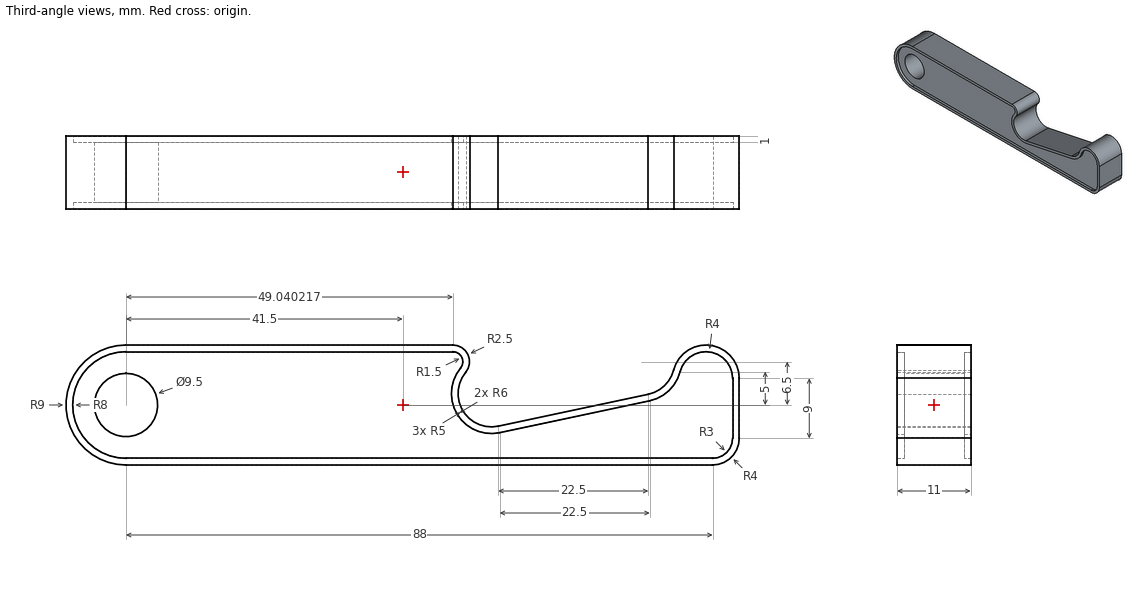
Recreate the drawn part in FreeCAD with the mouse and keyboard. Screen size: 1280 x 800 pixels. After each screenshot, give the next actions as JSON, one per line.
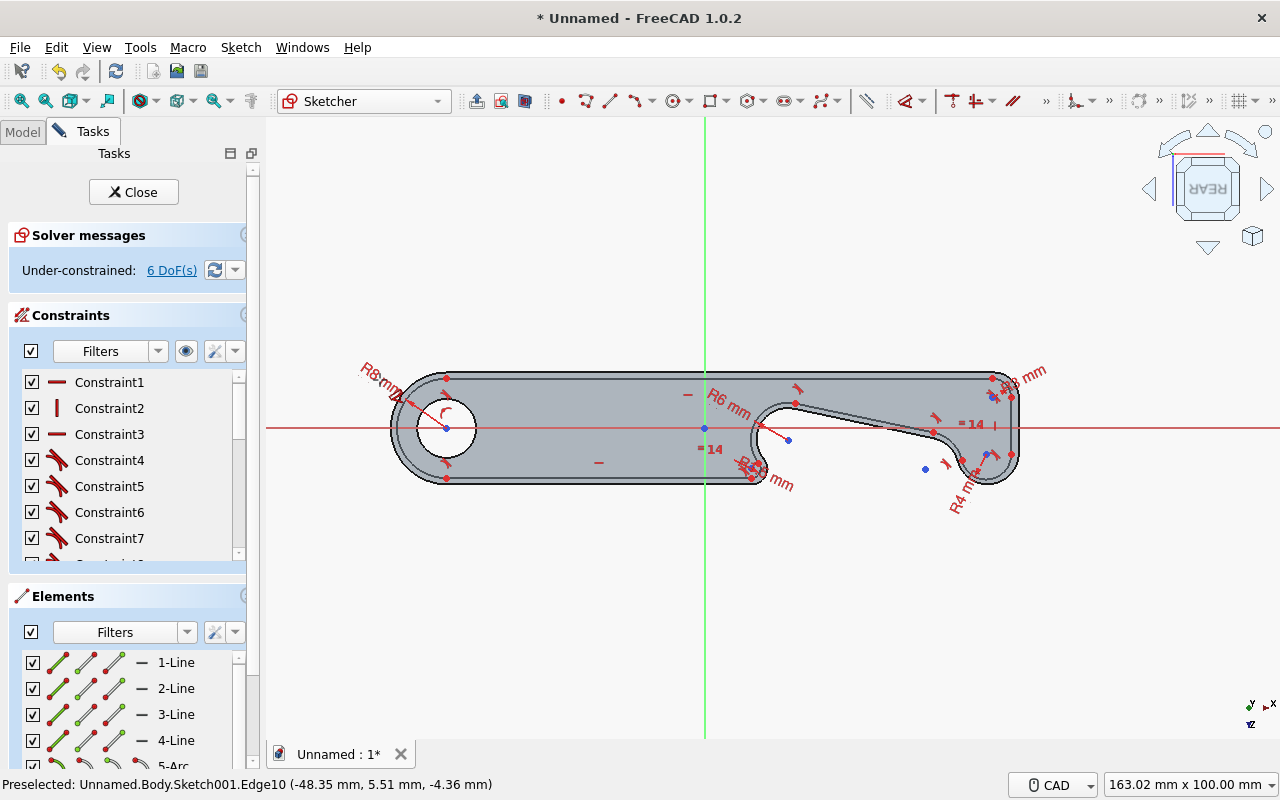
{"action": "scroll", "coordinate": [1011, 437], "scroll_direction": "up", "scroll_amount": 3}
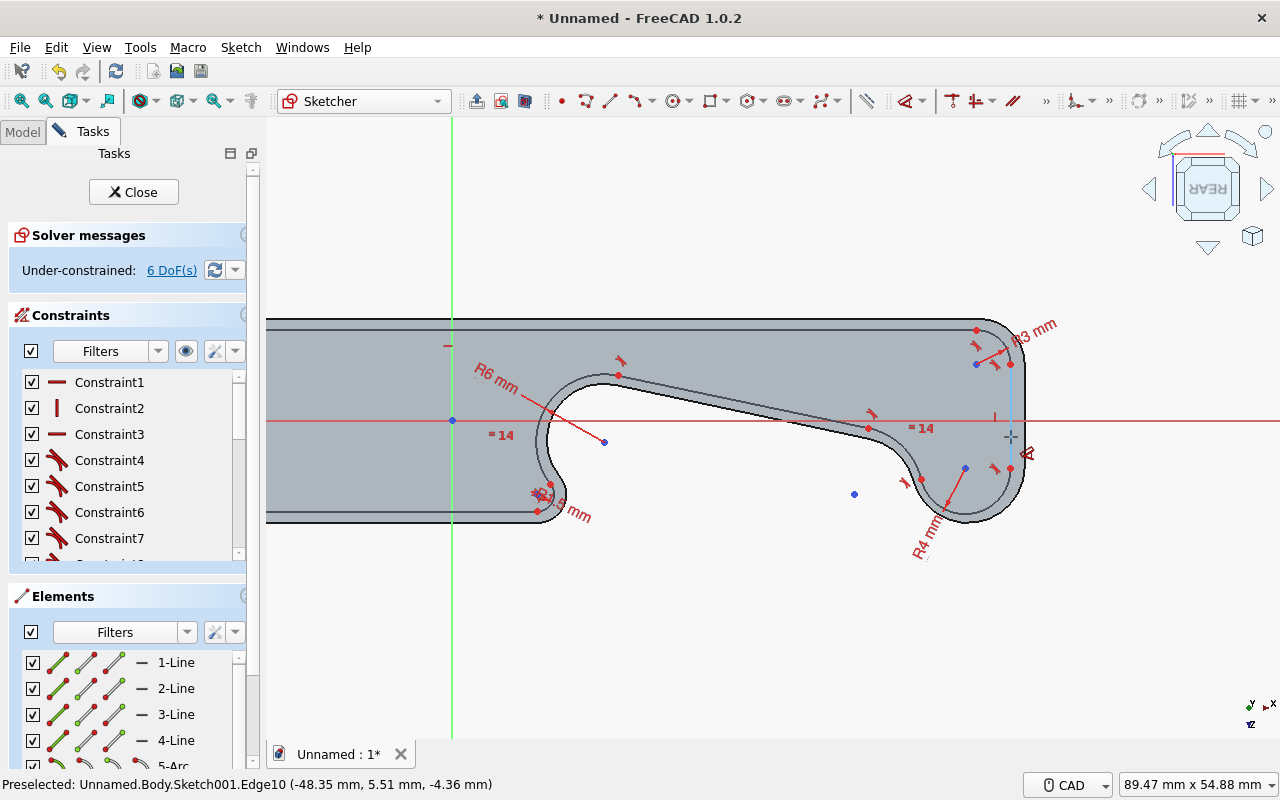
{"action": "left_click", "coordinate": [1011, 437]}
{"action": "left_click", "coordinate": [1045, 392]}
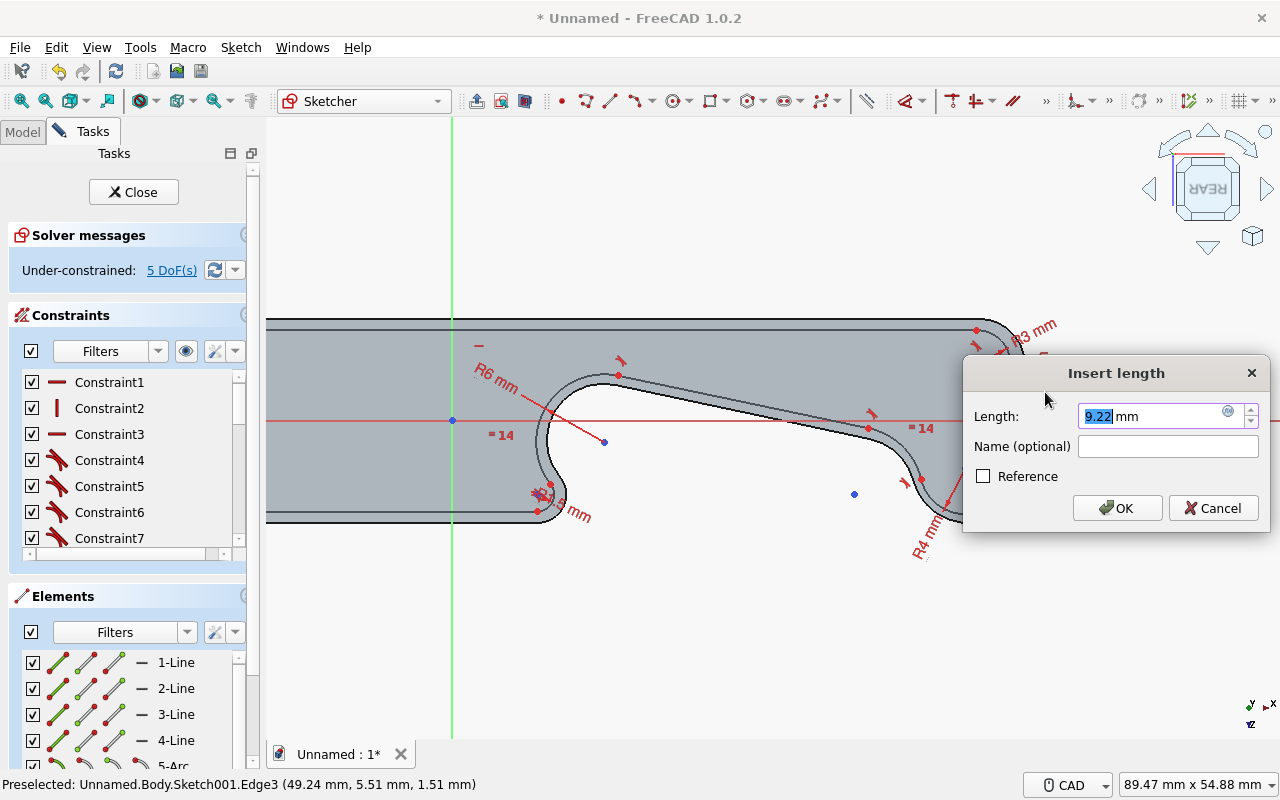
{"action": "type", "text": "9"}
{"action": "key", "text": "Return"}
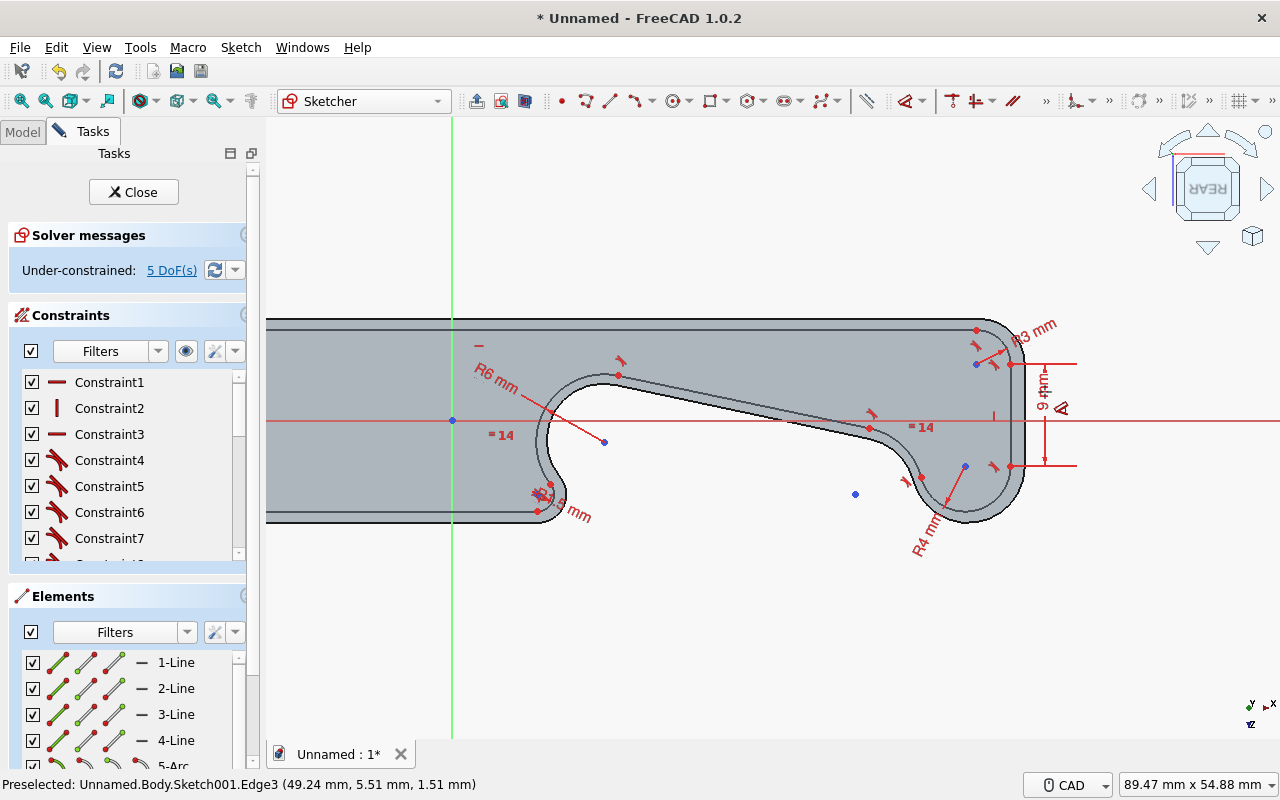
{"action": "left_click", "coordinate": [678, 330]}
{"action": "left_click", "coordinate": [635, 296]}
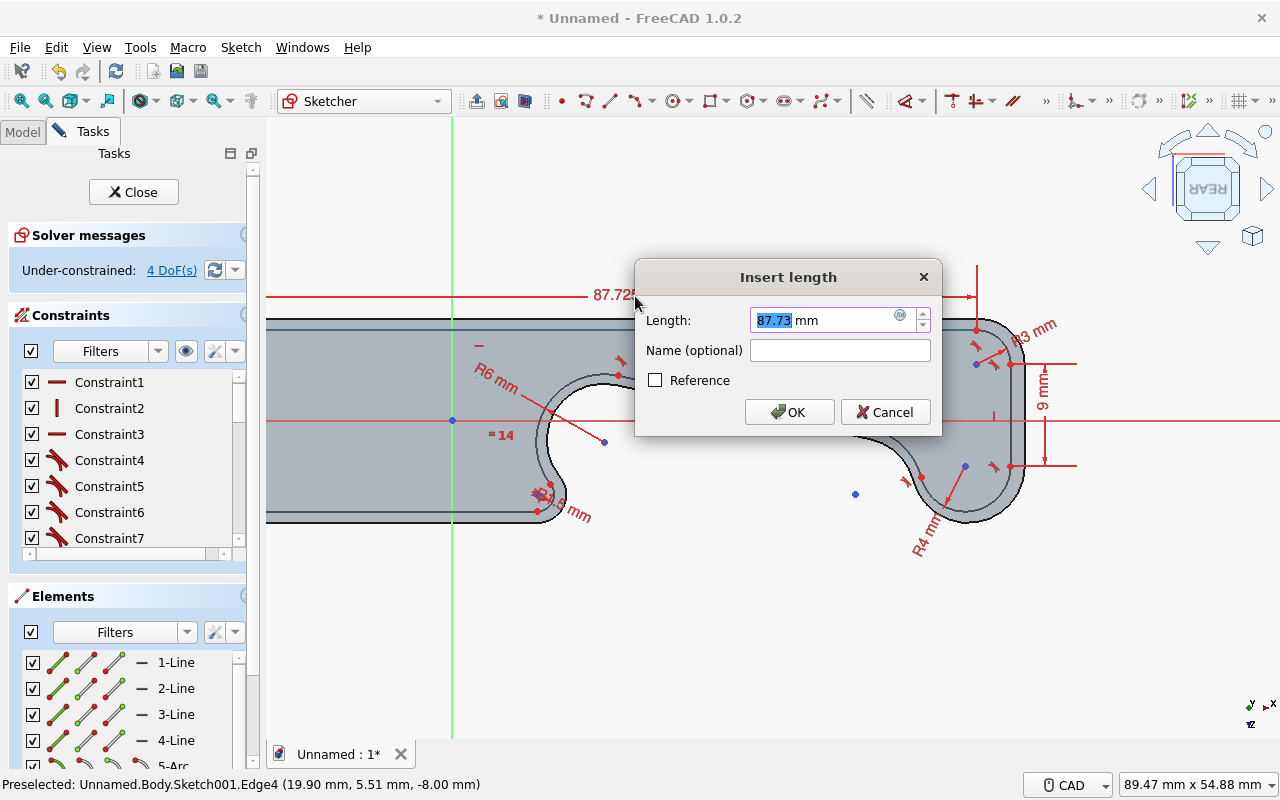
{"action": "type", "text": "88"}
{"action": "key", "text": "Return"}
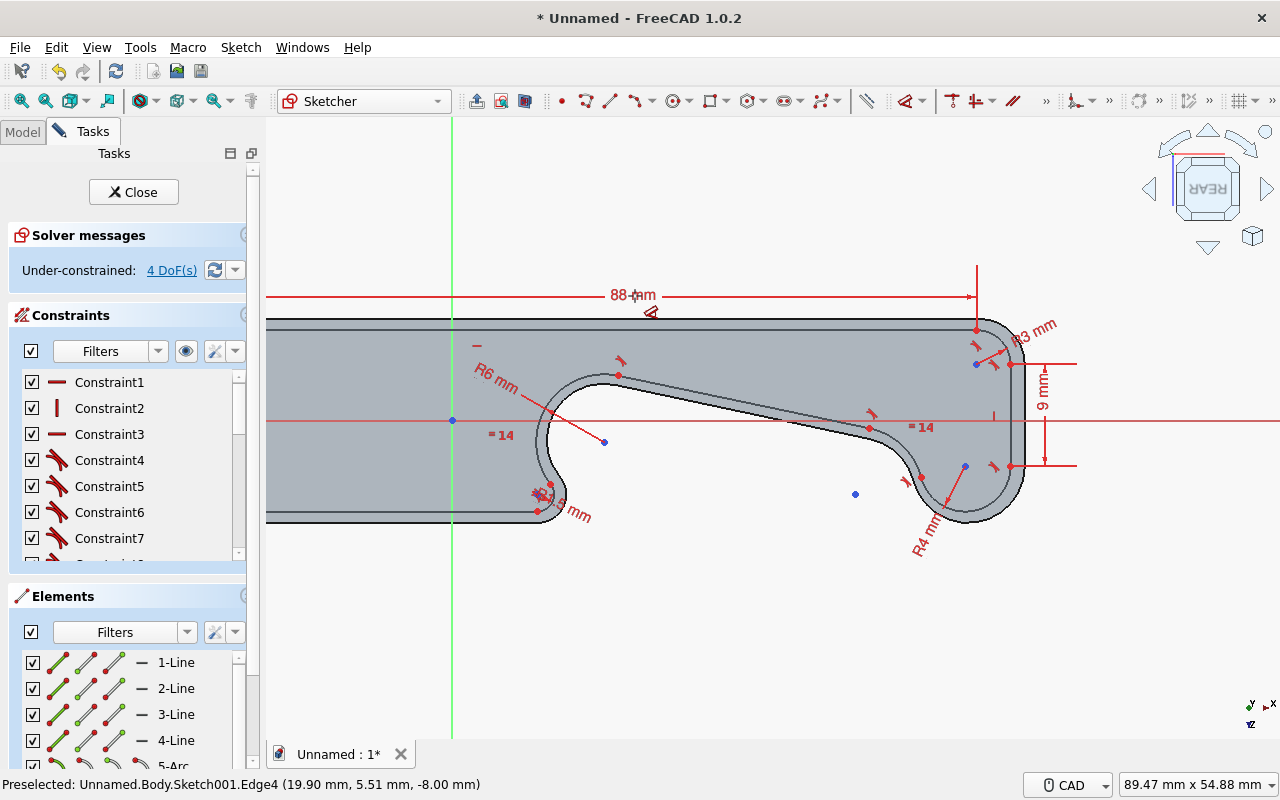
{"action": "left_click", "coordinate": [921, 478]}
{"action": "left_click", "coordinate": [955, 449]}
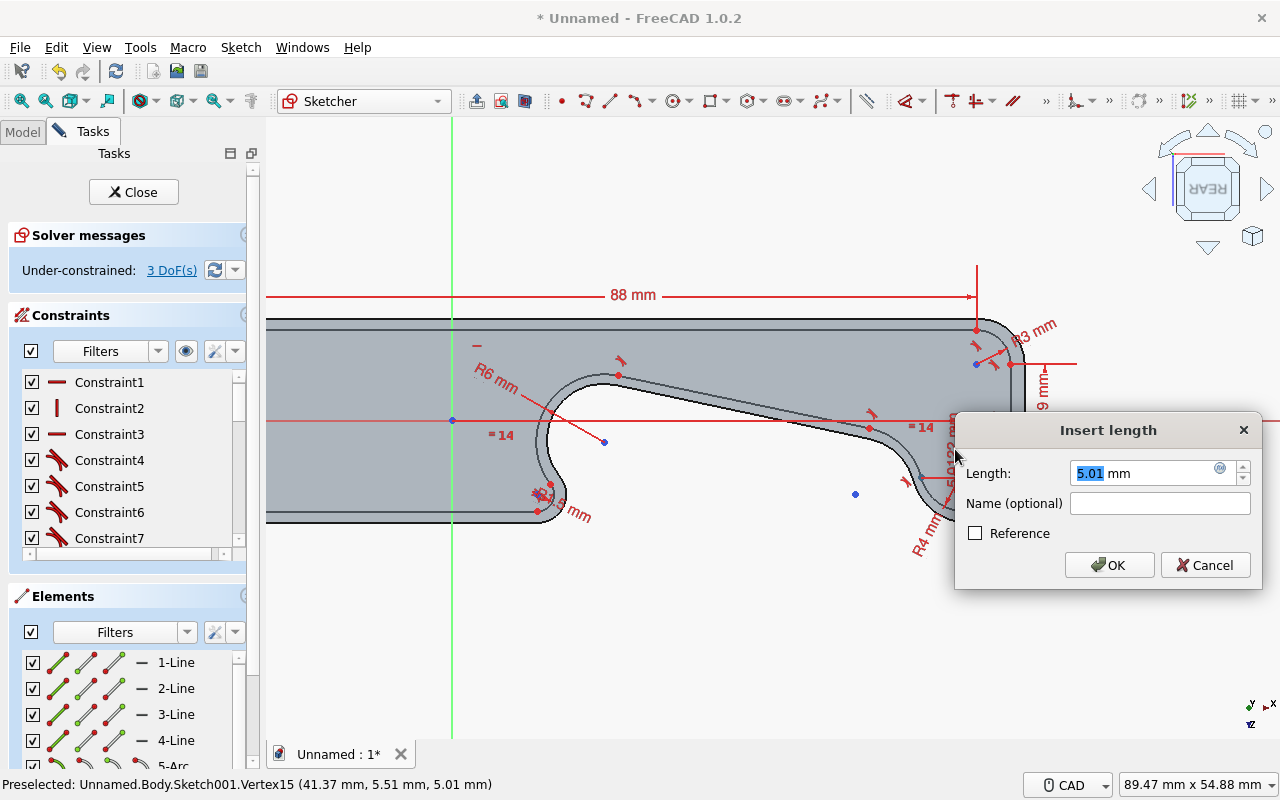
{"action": "type", "text": "5"}
{"action": "key", "text": "Return"}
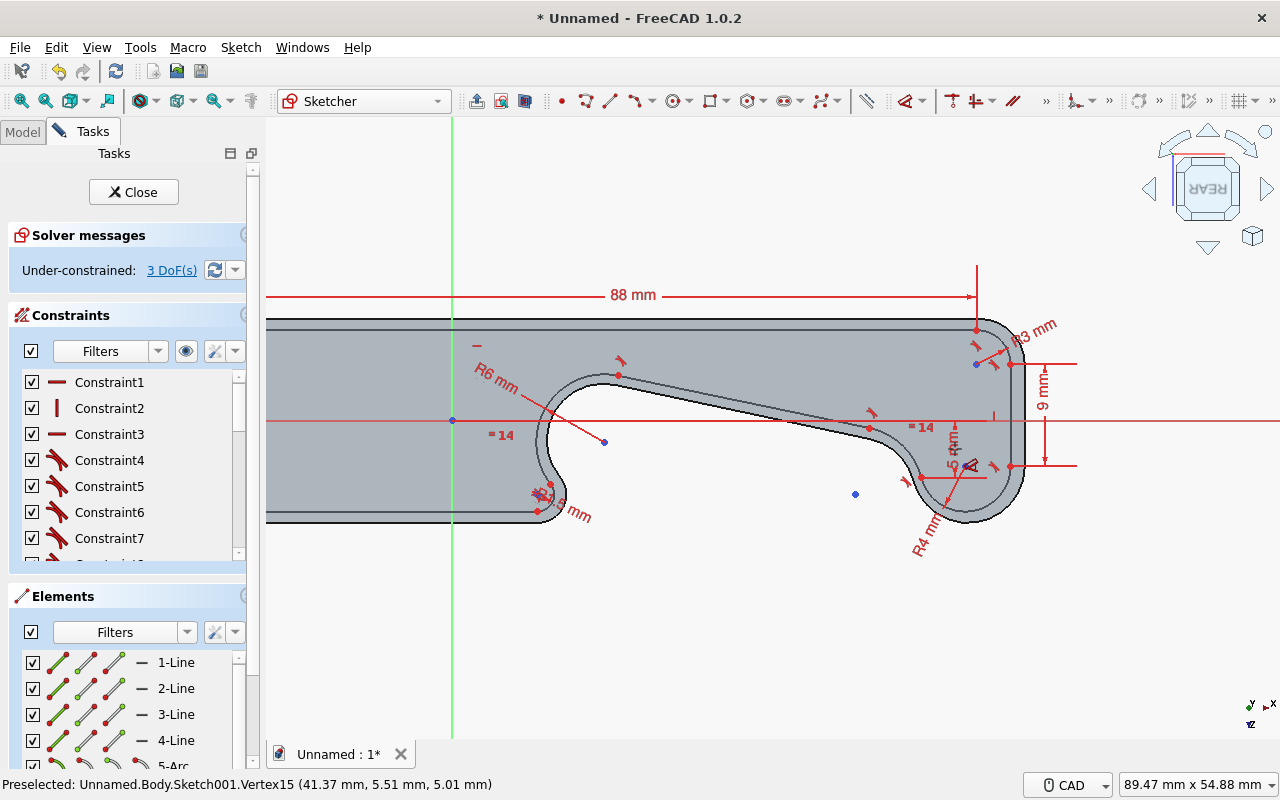
{"action": "scroll", "coordinate": [1011, 437], "scroll_direction": "down", "scroll_amount": 3}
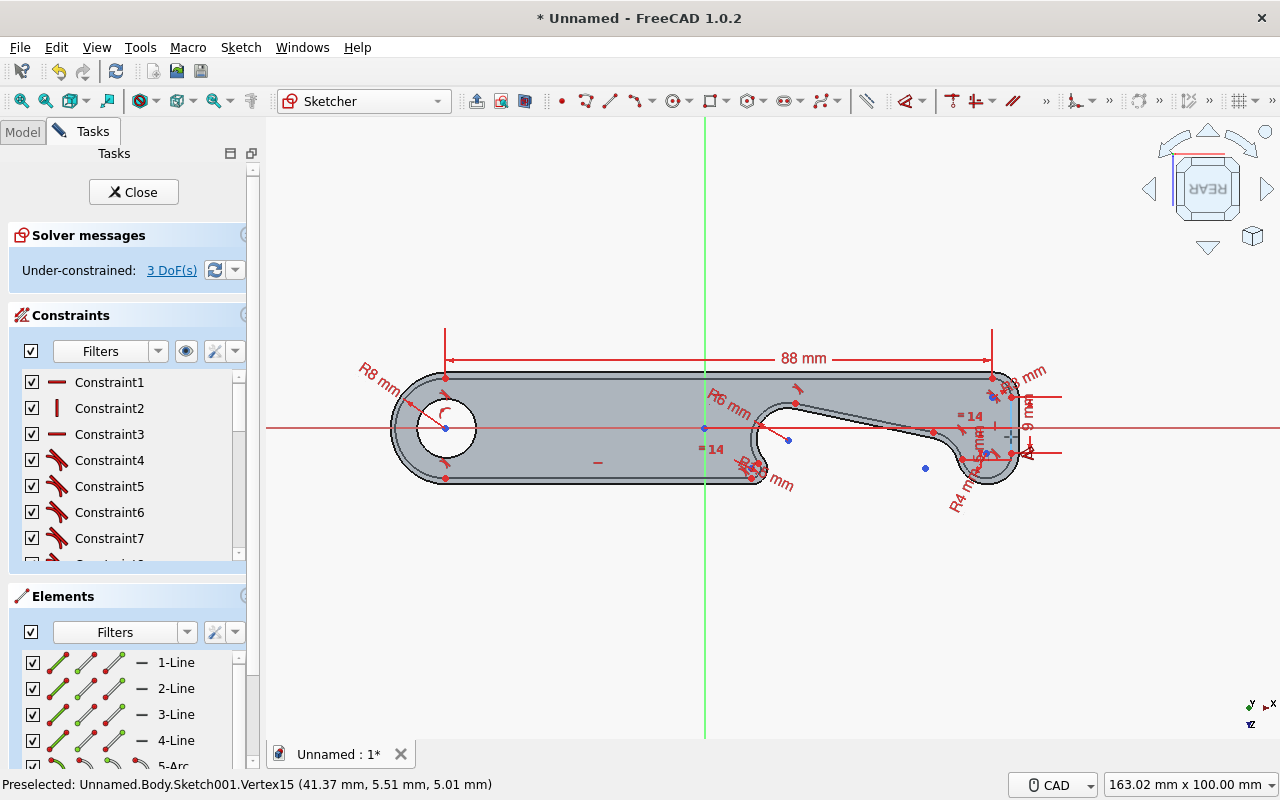
{"action": "left_click", "coordinate": [445, 478]}
{"action": "left_click", "coordinate": [575, 512]}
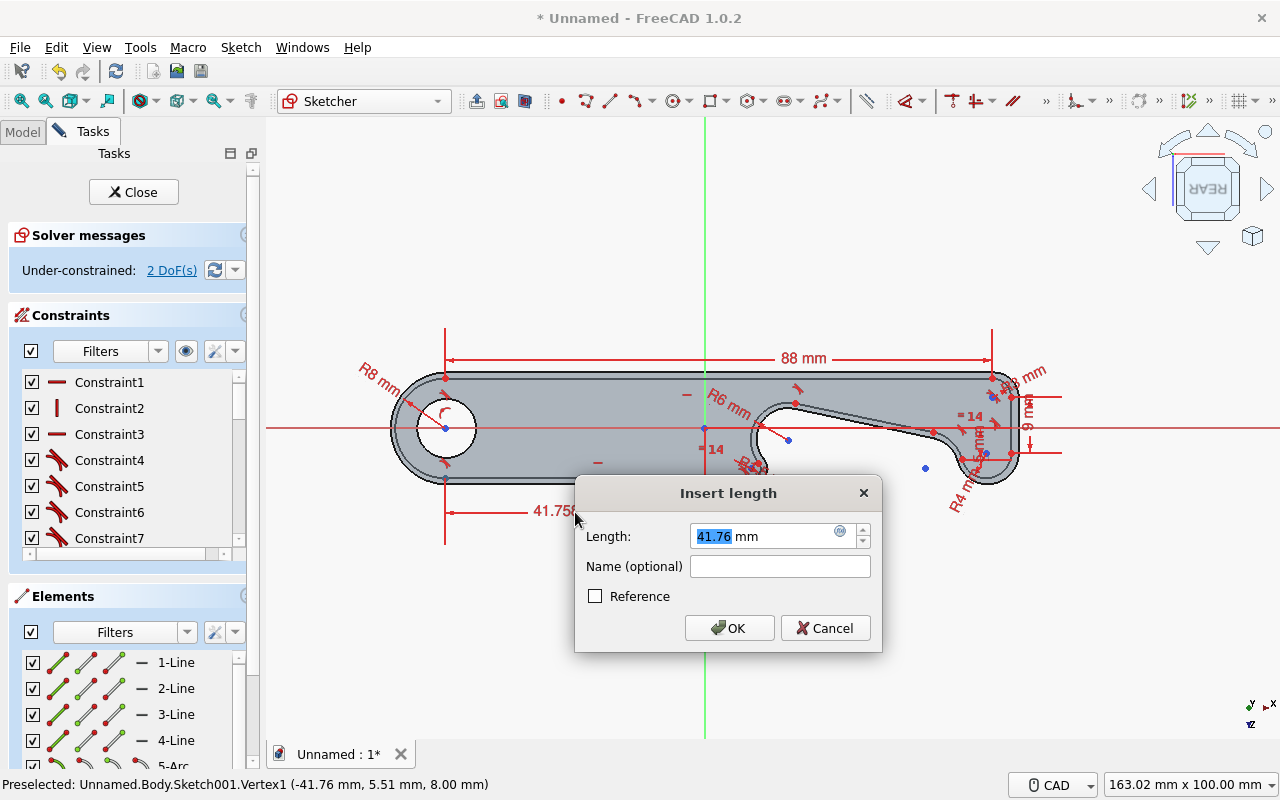
{"action": "type", "text": "41.5"}
{"action": "key", "text": "Return"}